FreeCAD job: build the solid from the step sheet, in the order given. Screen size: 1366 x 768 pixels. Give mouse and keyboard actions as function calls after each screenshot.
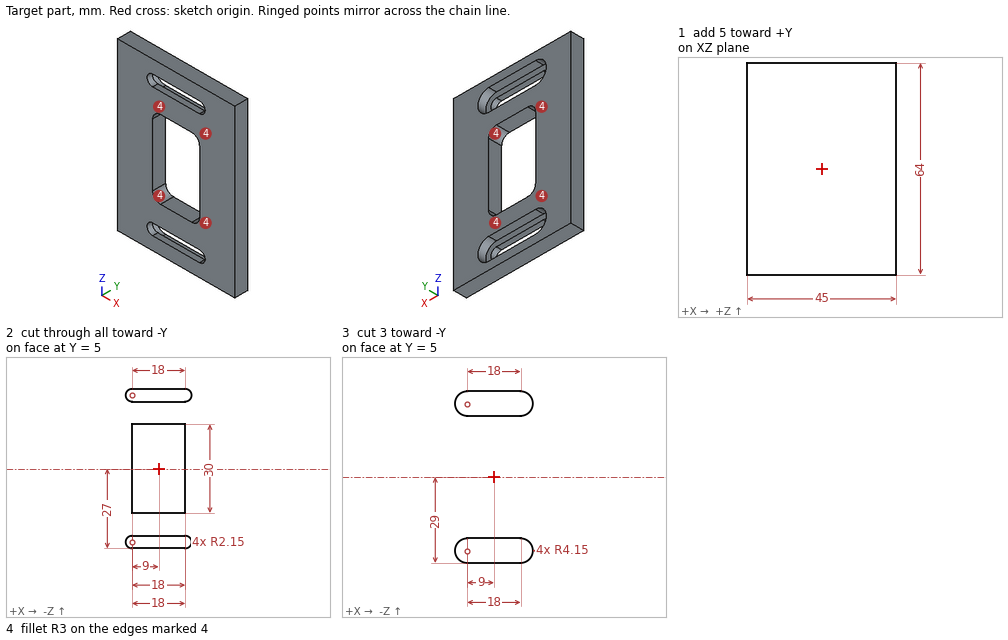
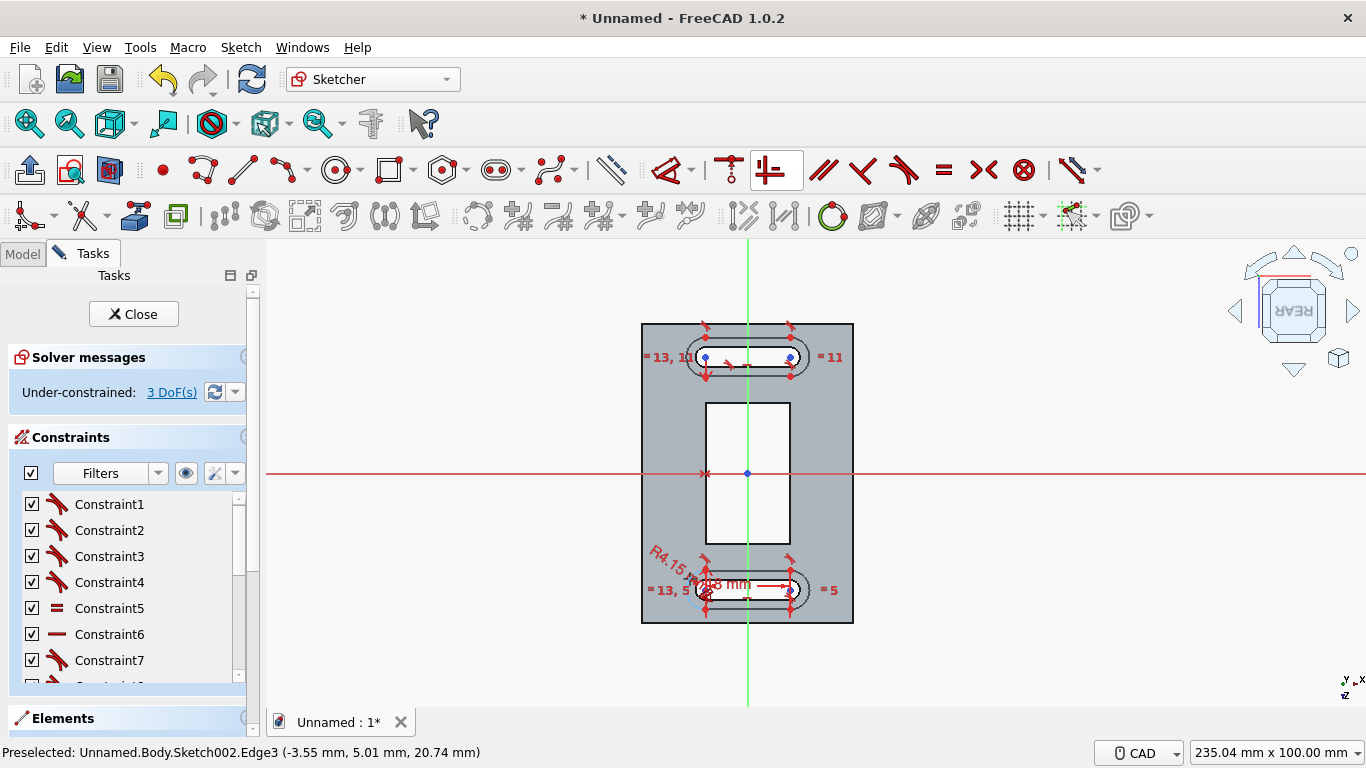
click(731, 338)
click(729, 304)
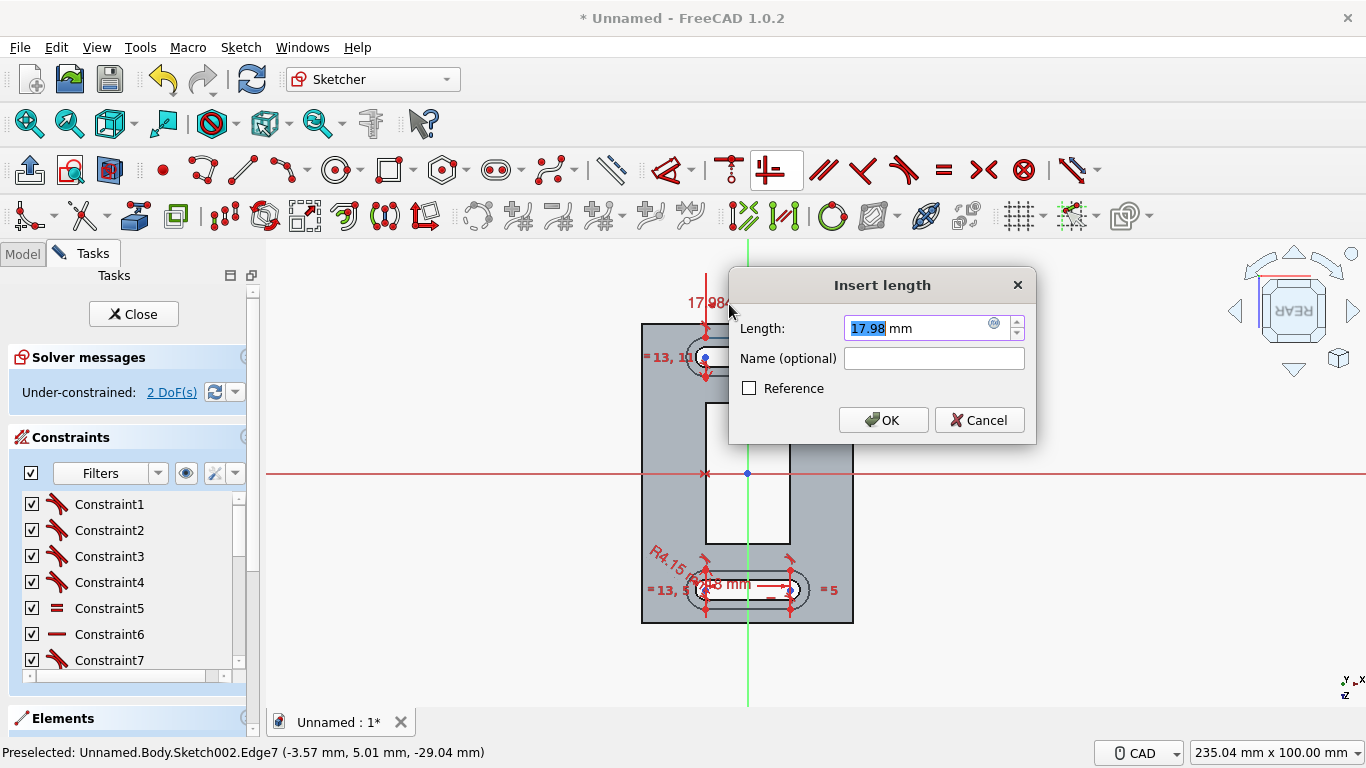
text(18)
key(Return)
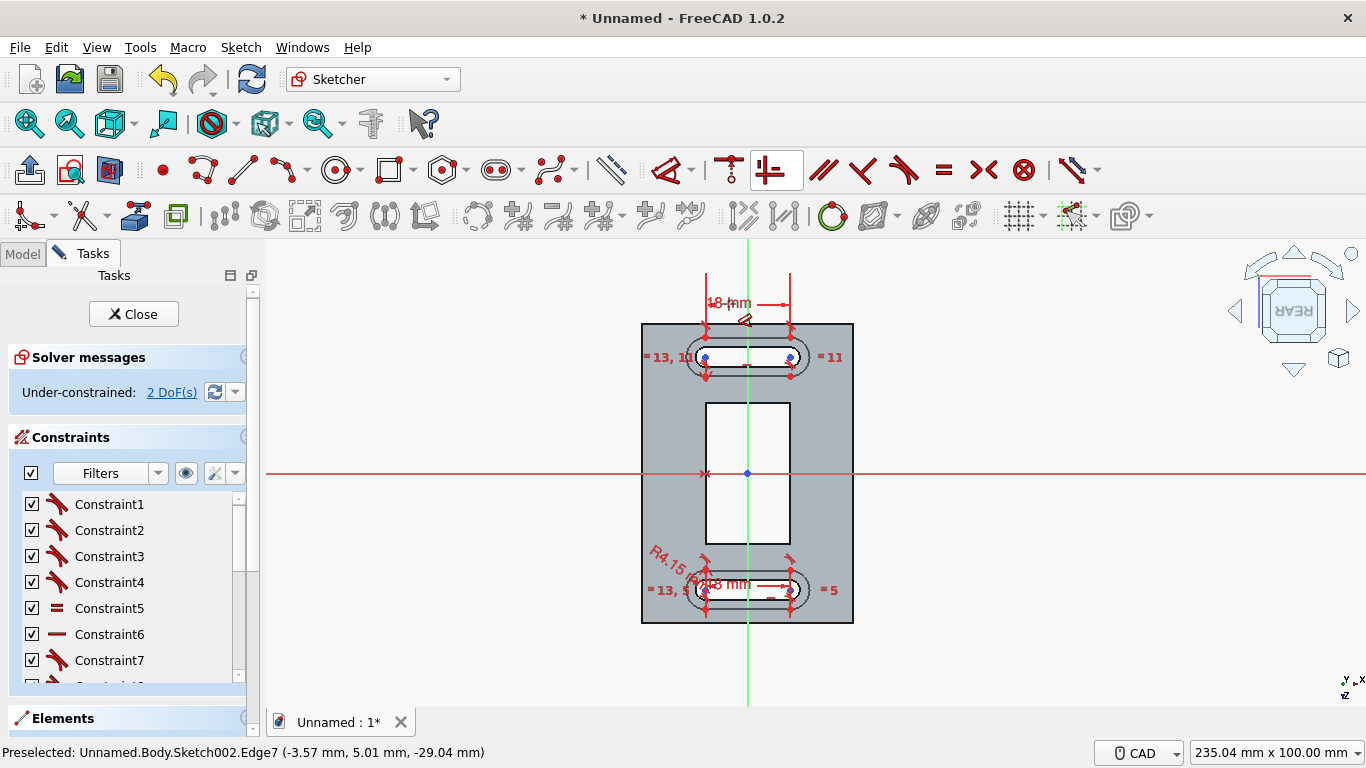
click(706, 571)
click(727, 440)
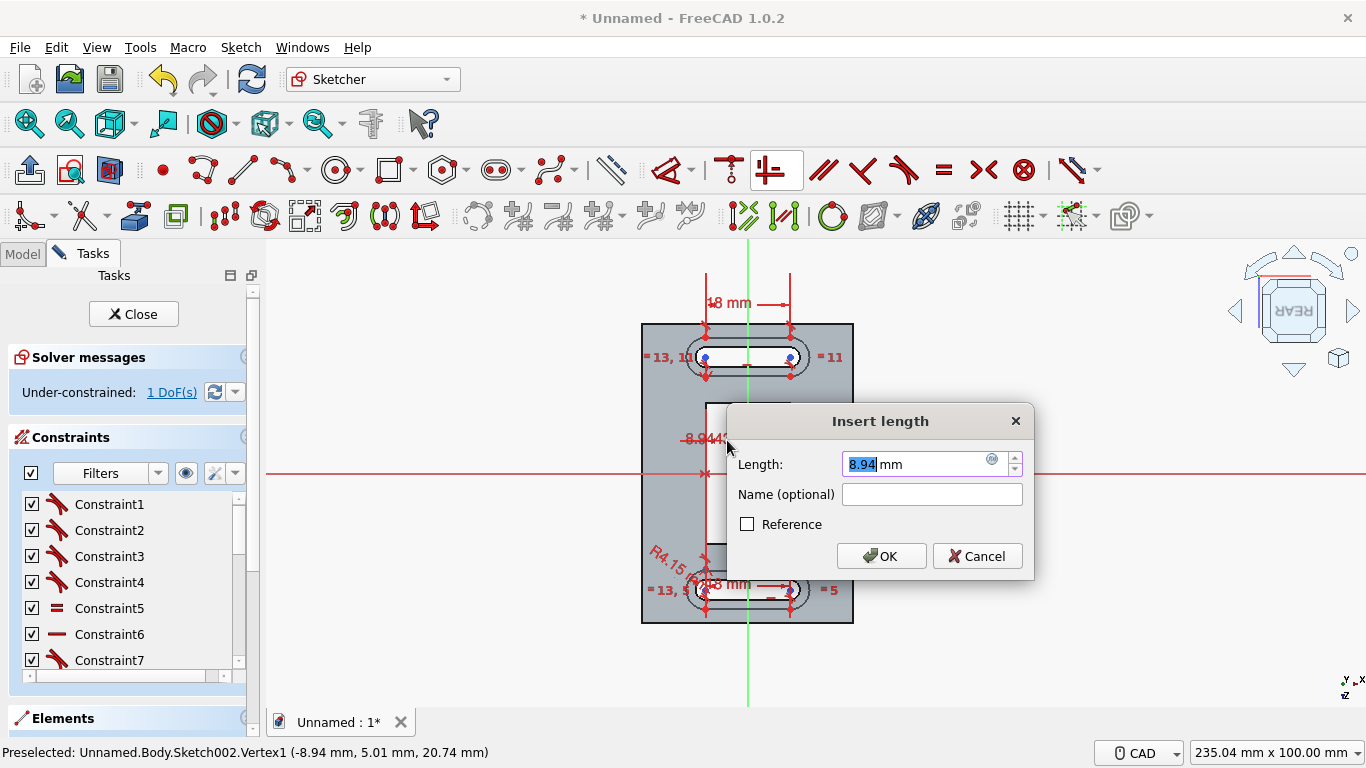
text(9)
key(Return)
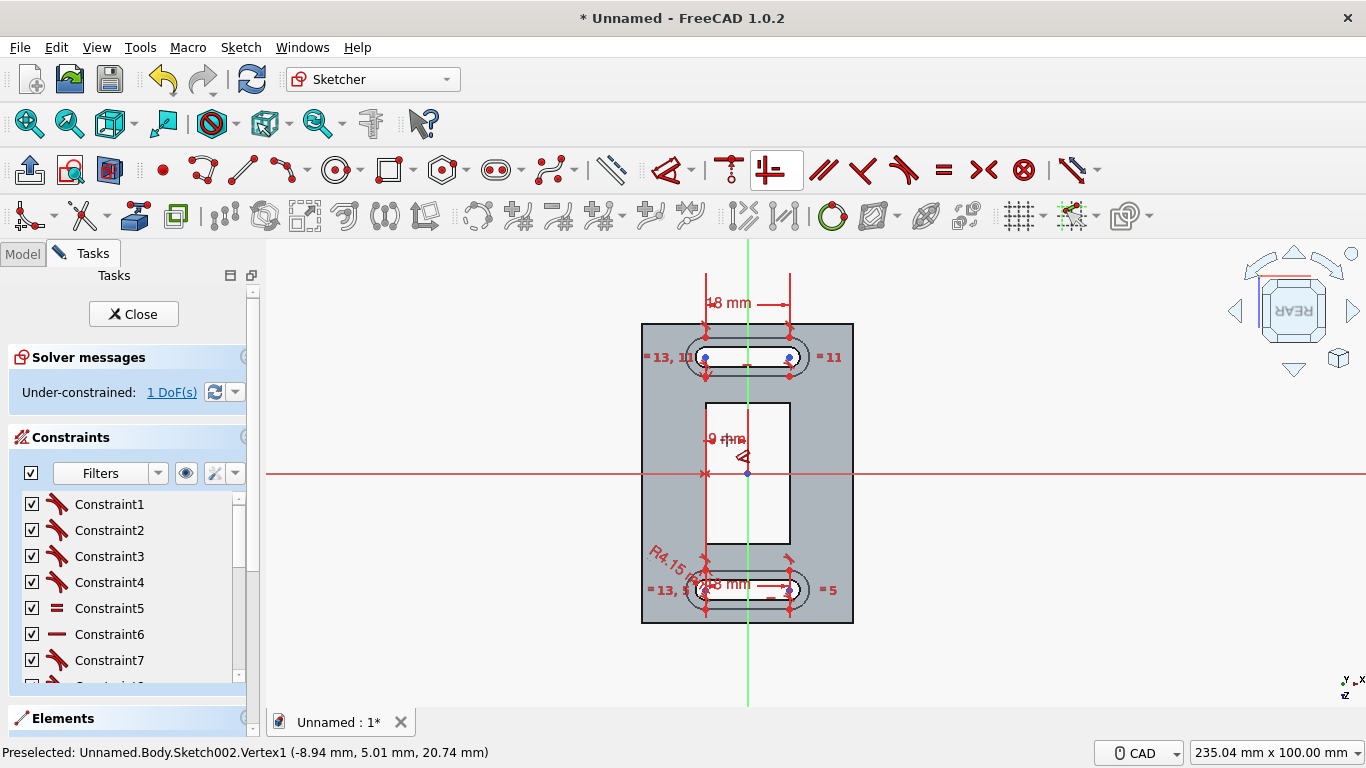
click(706, 609)
click(672, 542)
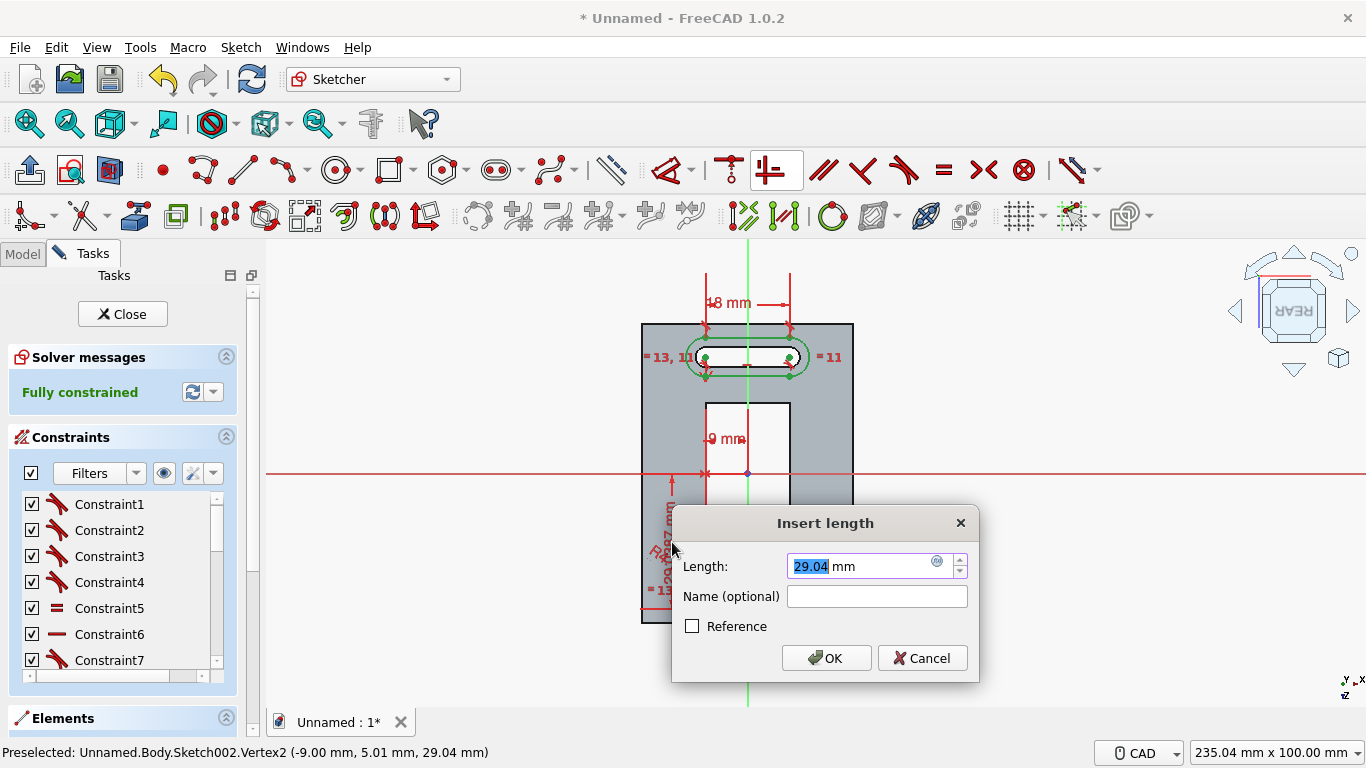
text(29)
key(Return)
key(Escape)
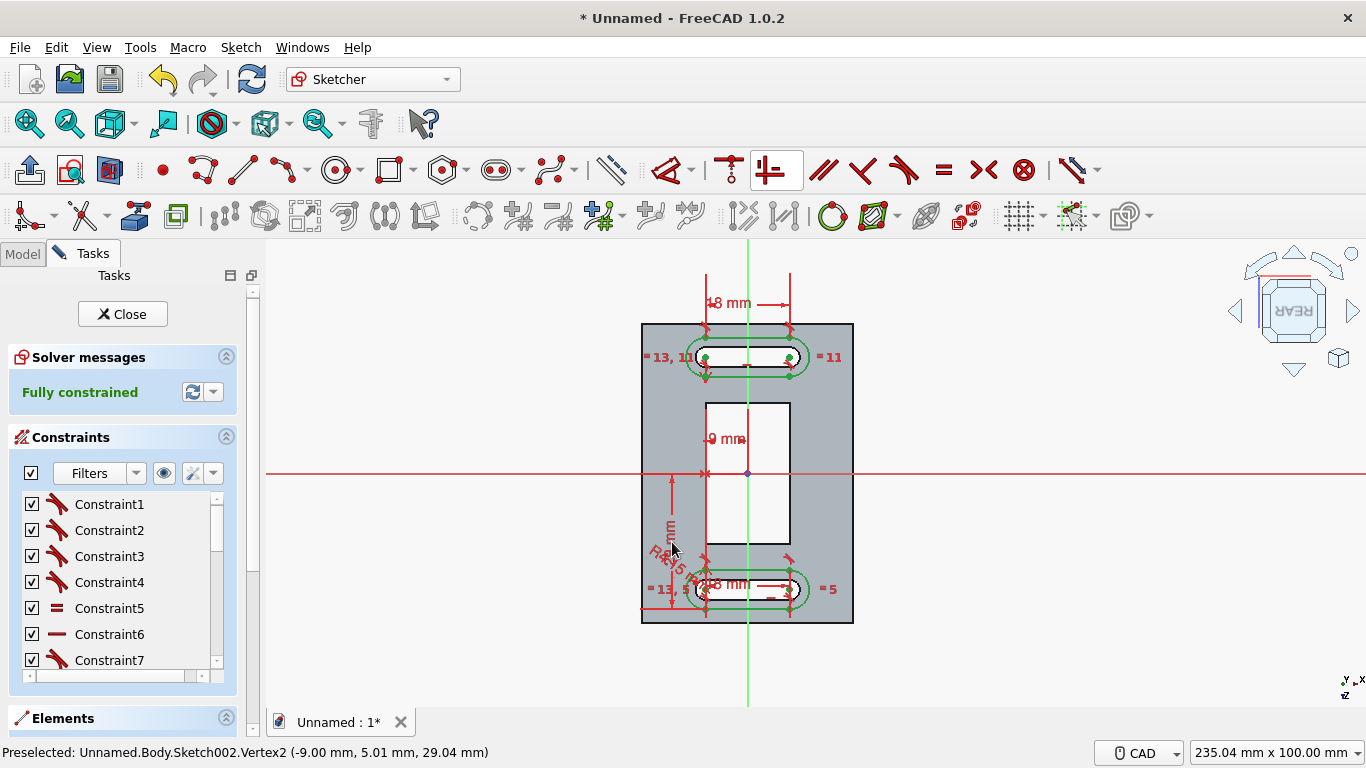
click(123, 314)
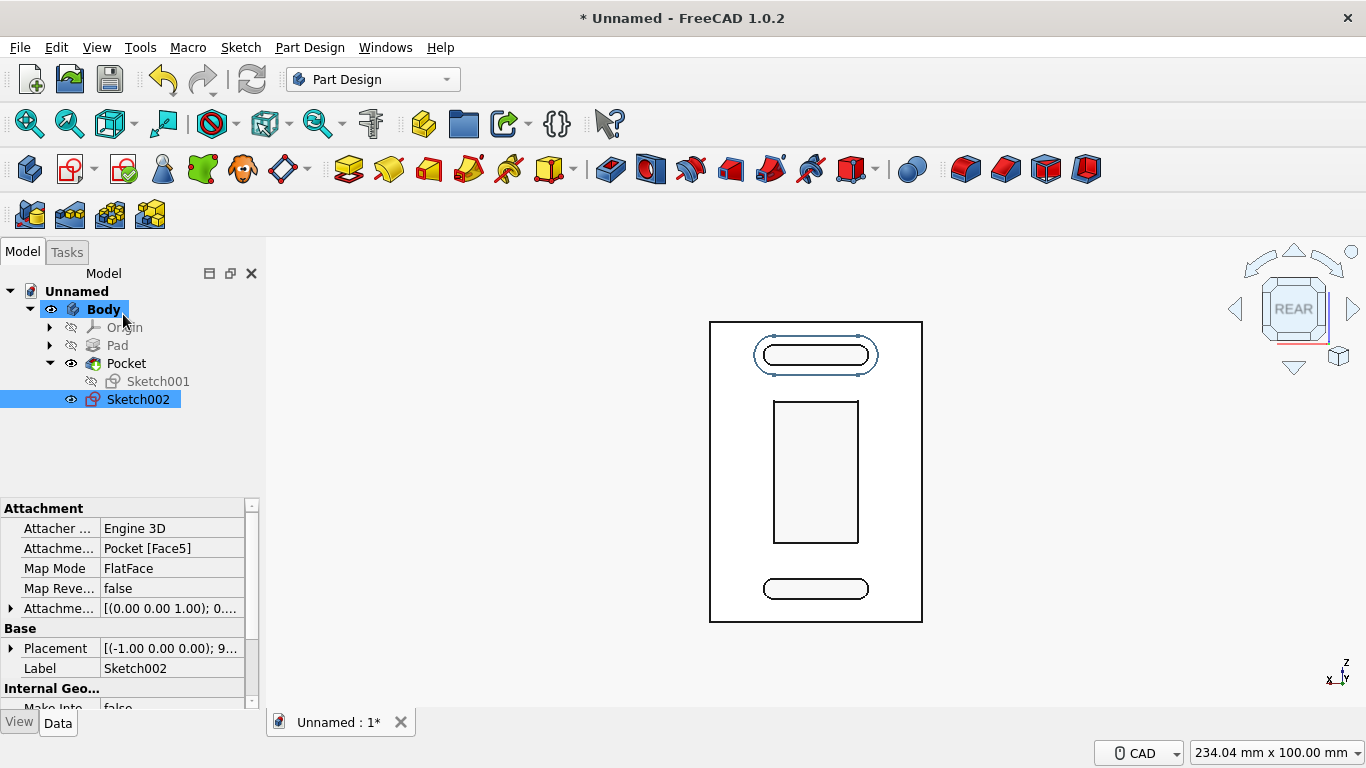
click(612, 170)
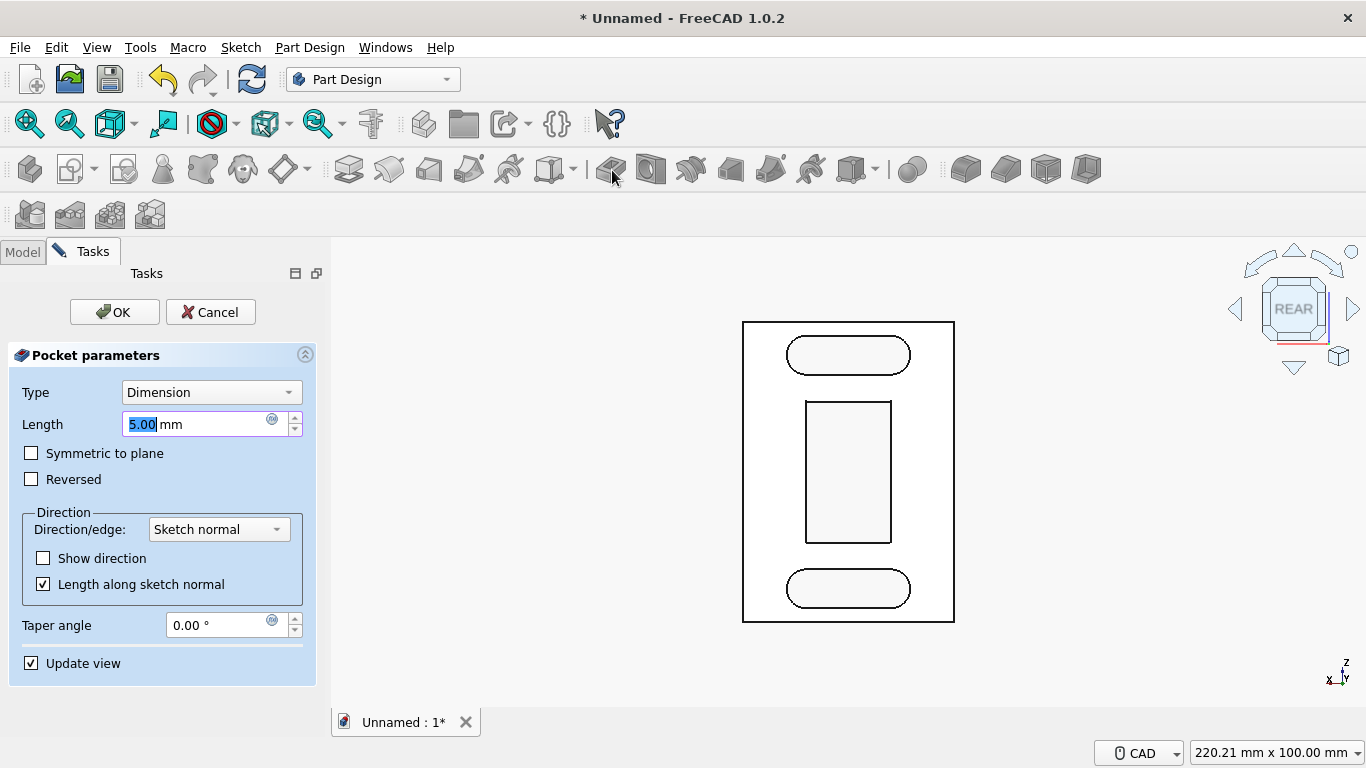
text(3)
key(Tab)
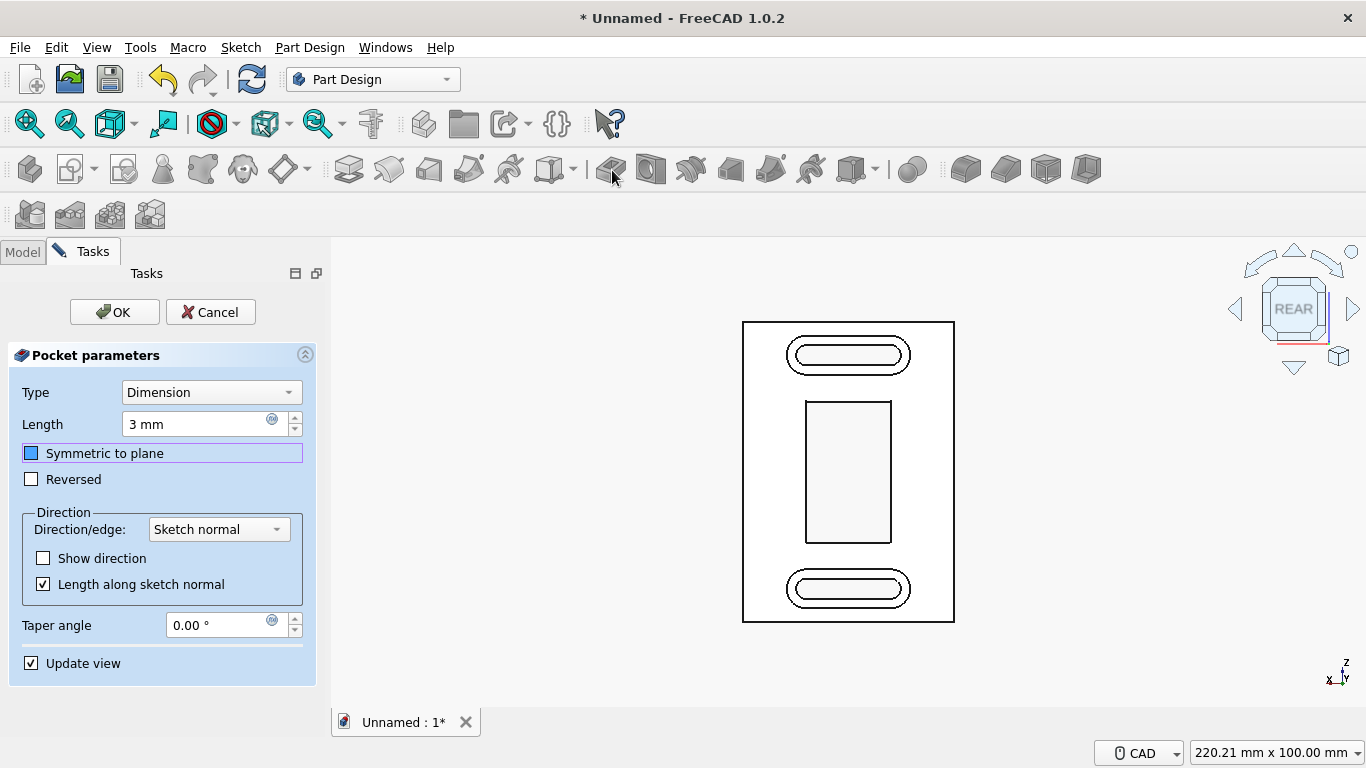
click(115, 312)